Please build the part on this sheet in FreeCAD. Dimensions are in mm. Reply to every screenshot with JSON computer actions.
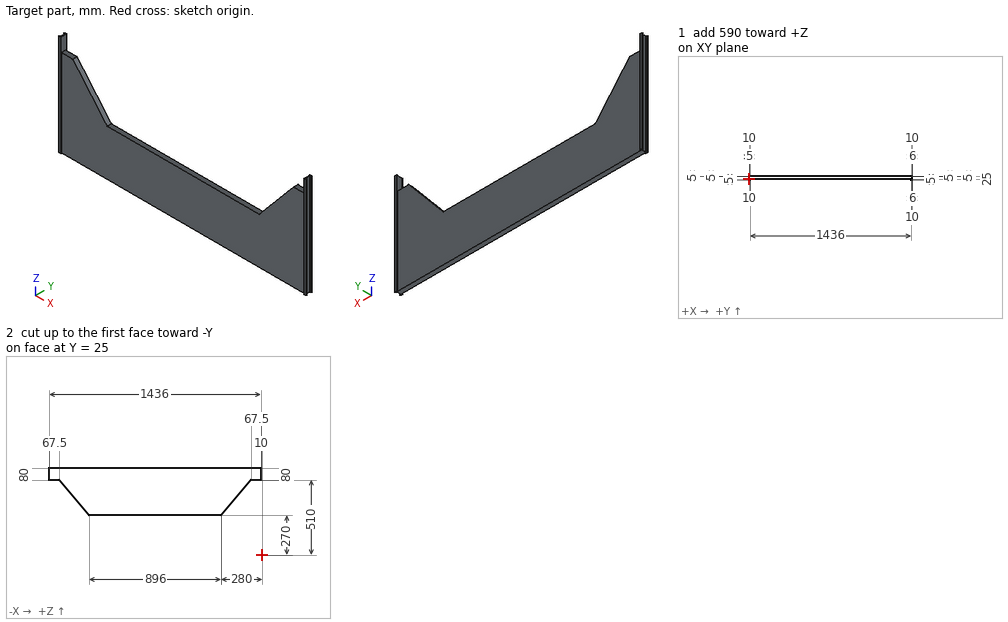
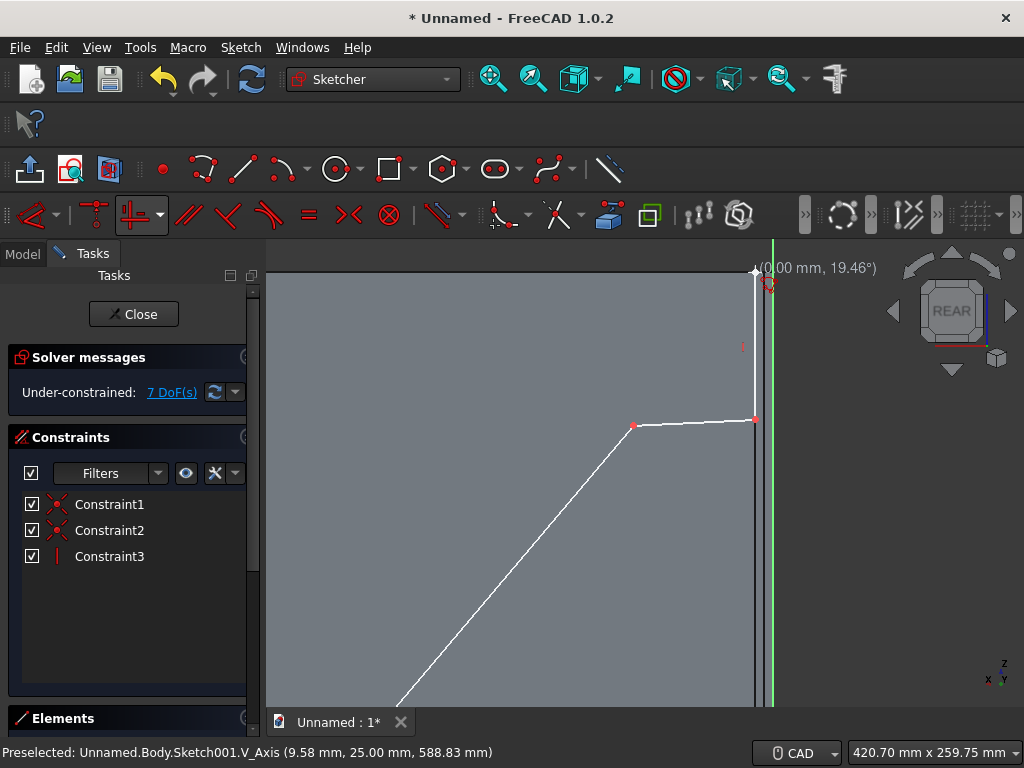
{"action": "scroll", "coordinate": [796, 408], "scroll_direction": "down", "scroll_amount": 9}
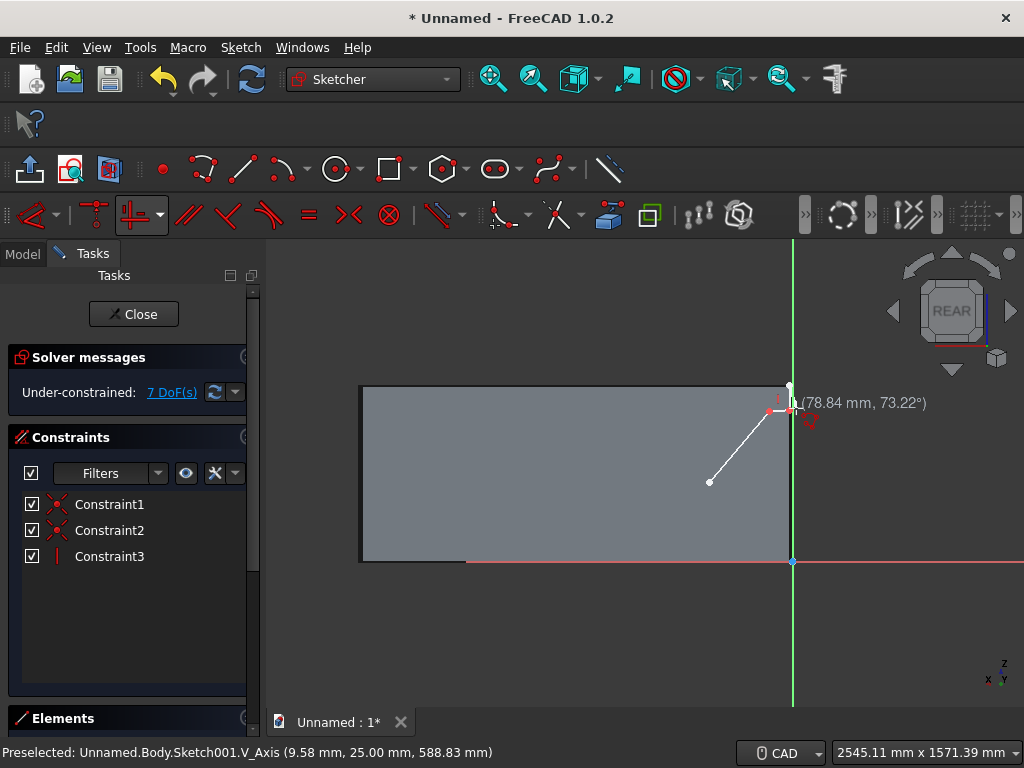
{"action": "left_click", "coordinate": [362, 386]}
{"action": "left_click", "coordinate": [362, 410]}
{"action": "left_click", "coordinate": [382, 410]}
{"action": "left_click", "coordinate": [443, 481]}
{"action": "left_click", "coordinate": [710, 482]}
{"action": "key", "text": "Escape"}
{"action": "key", "text": "Escape"}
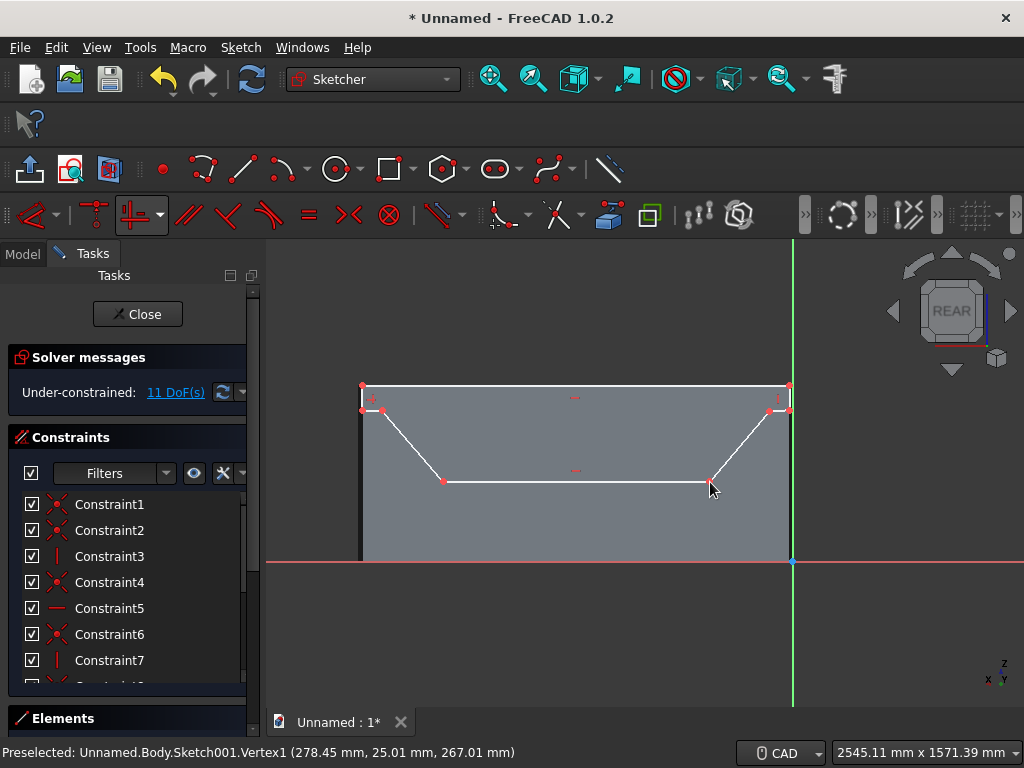
{"action": "scroll", "coordinate": [780, 411], "scroll_direction": "up", "scroll_amount": 2}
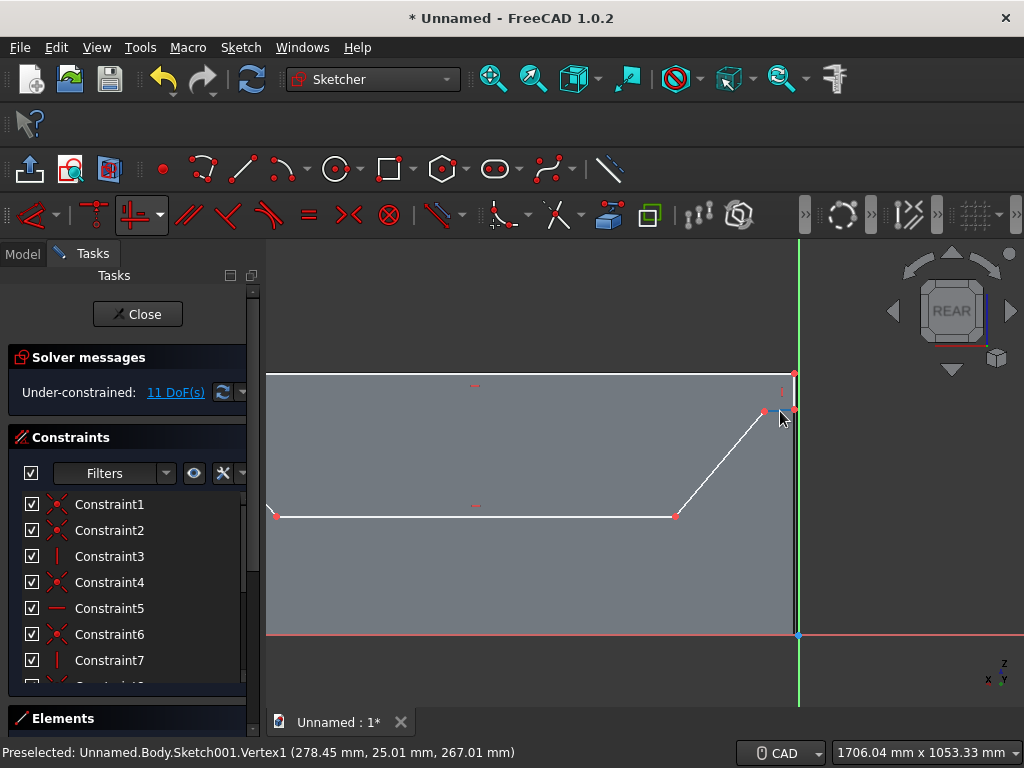
{"action": "left_click", "coordinate": [779, 410]}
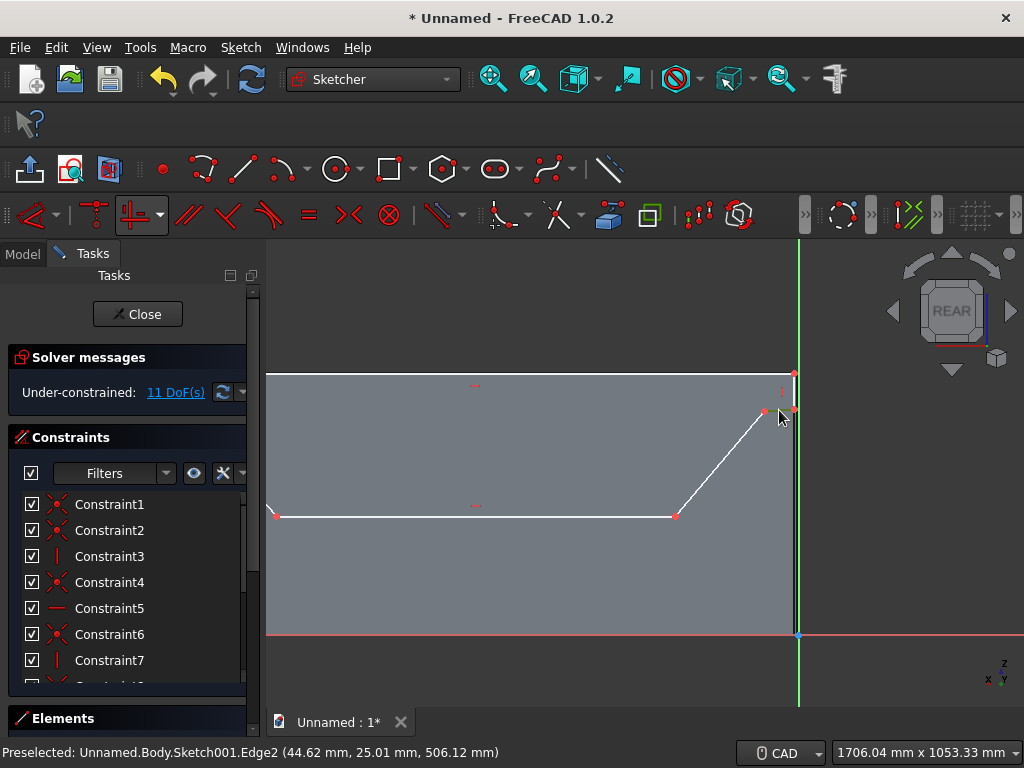
{"action": "key", "text": "h"}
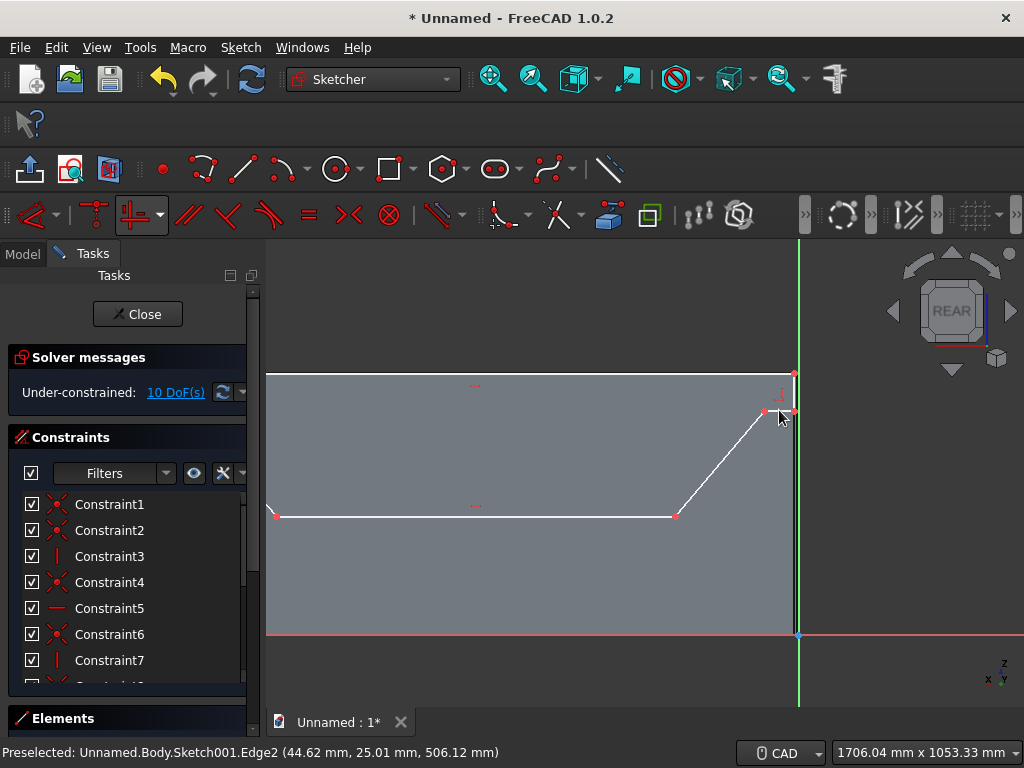
{"action": "left_click", "coordinate": [32, 216]}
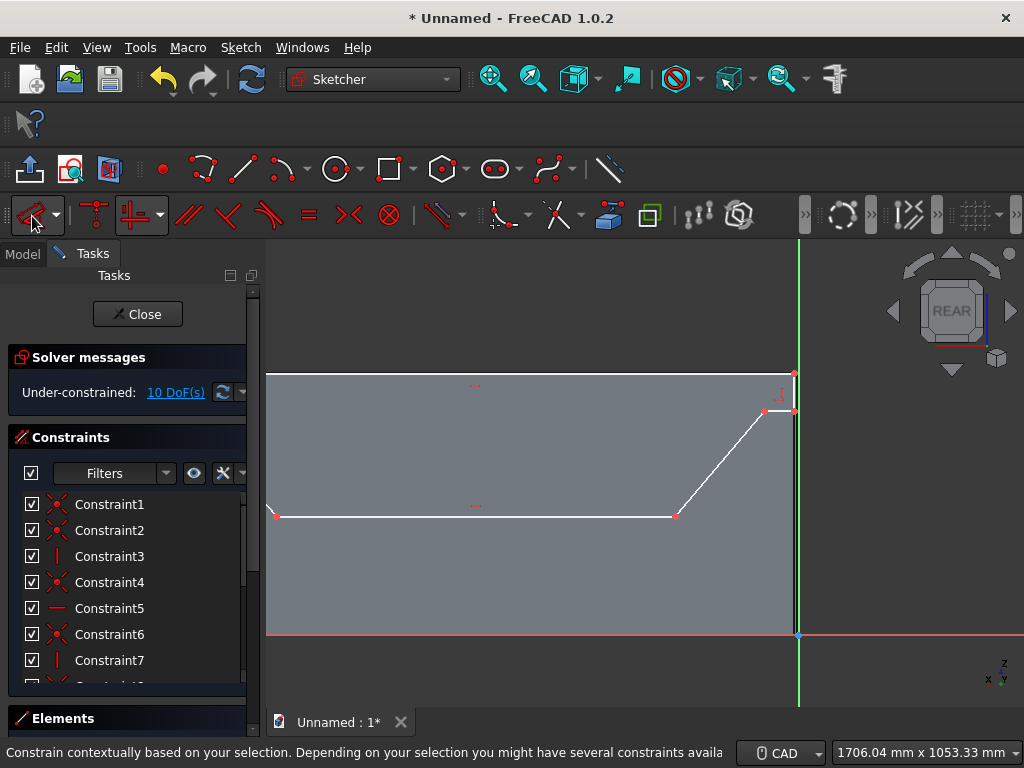
{"action": "scroll", "coordinate": [794, 400], "scroll_direction": "up", "scroll_amount": 6}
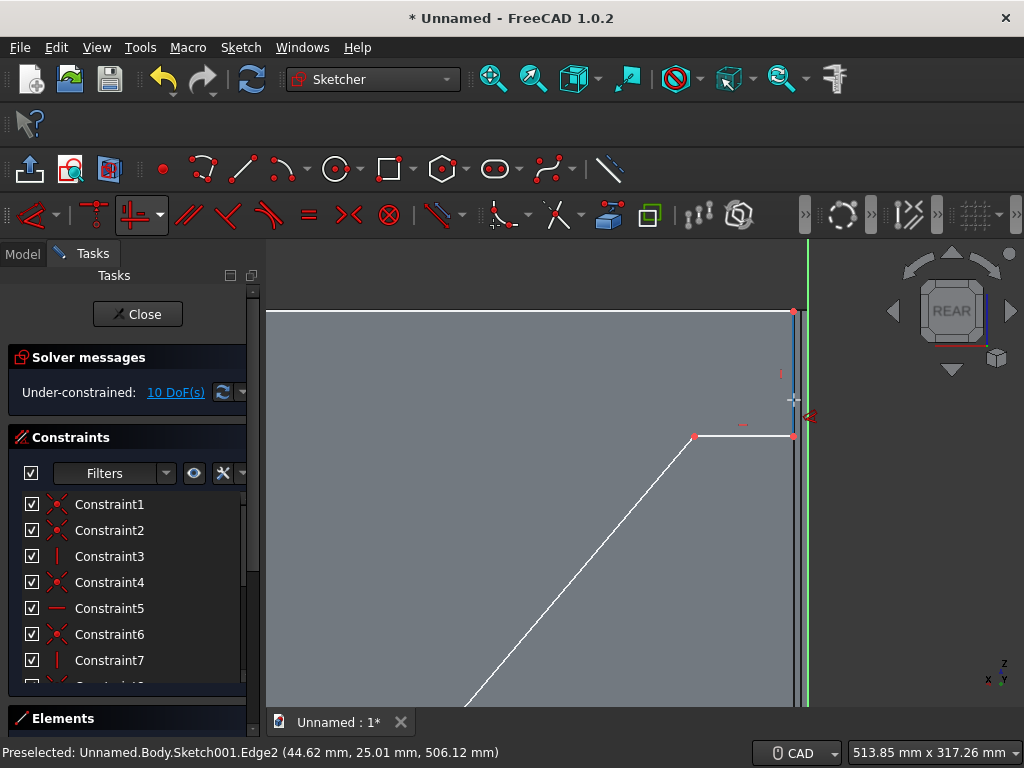
{"action": "left_click", "coordinate": [793, 399]}
{"action": "left_click", "coordinate": [827, 374]}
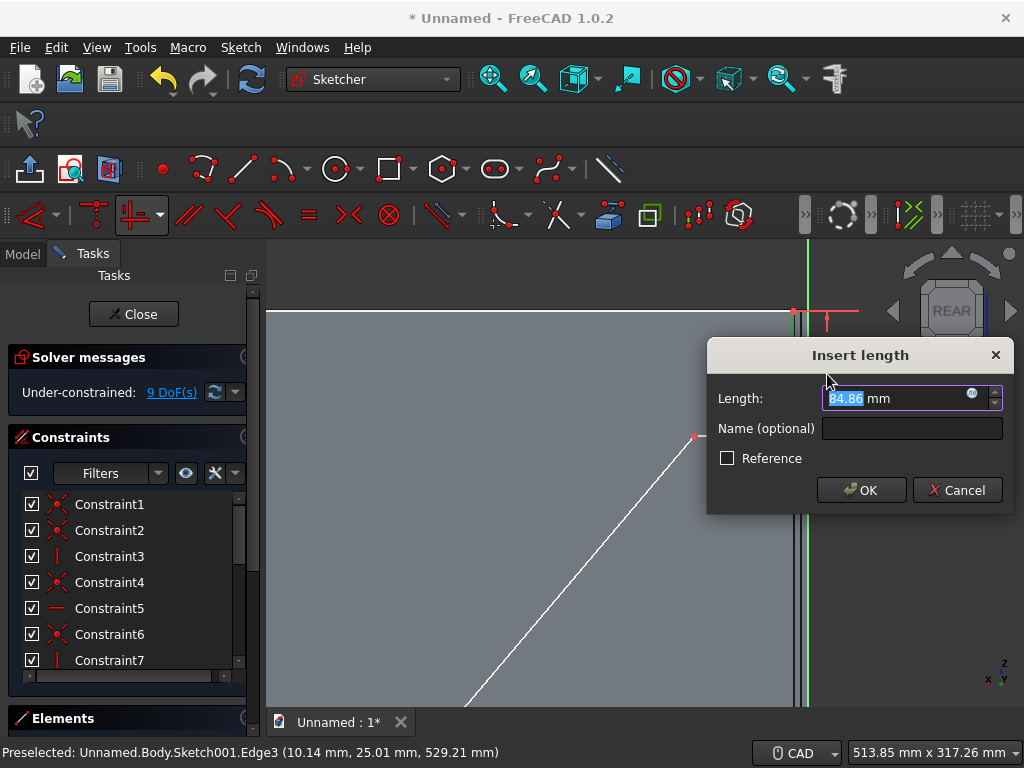
{"action": "type", "text": "80"}
{"action": "key", "text": "Return"}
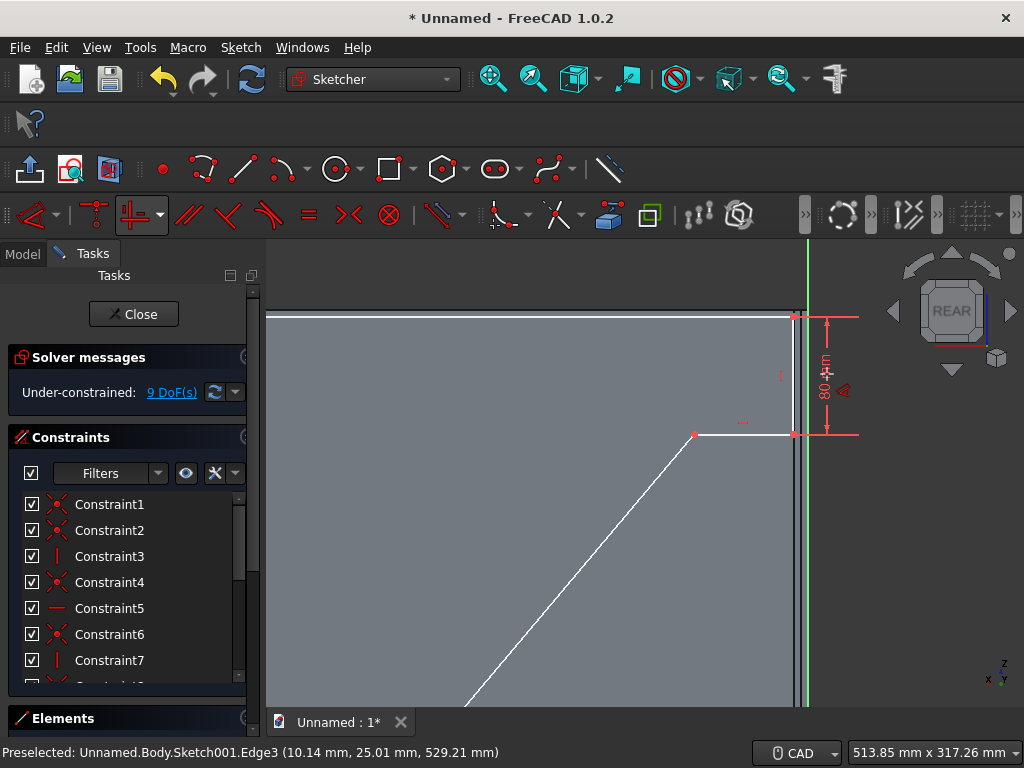
{"action": "scroll", "coordinate": [788, 404], "scroll_direction": "down", "scroll_amount": 8}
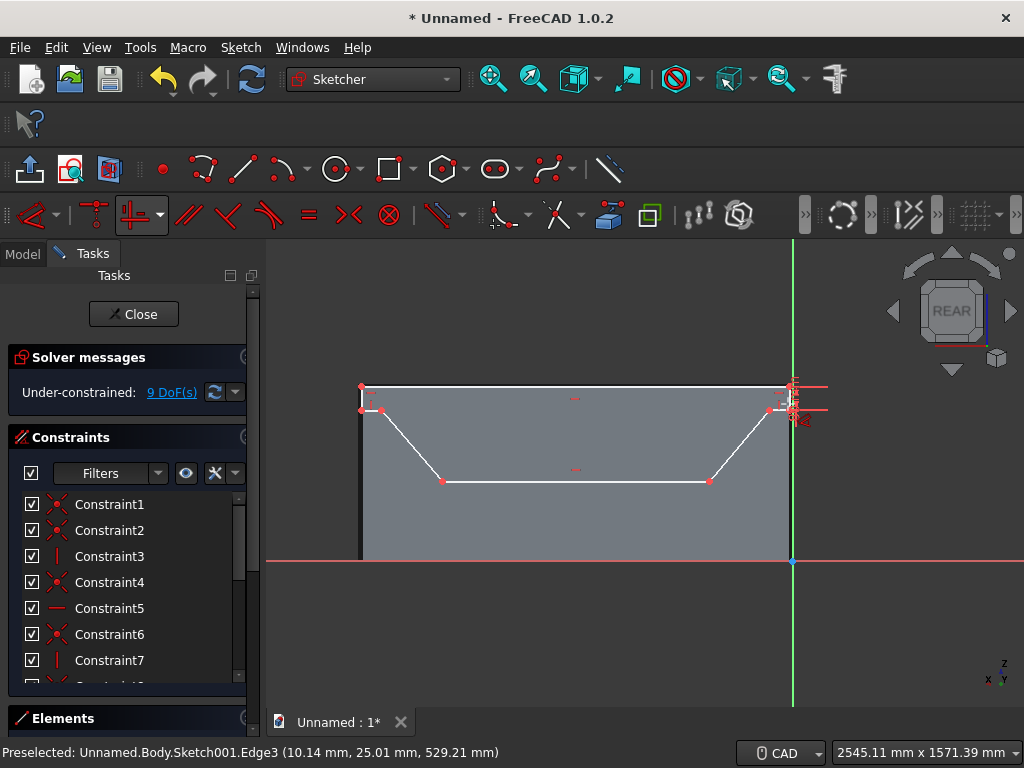
{"action": "scroll", "coordinate": [362, 394], "scroll_direction": "up", "scroll_amount": 4}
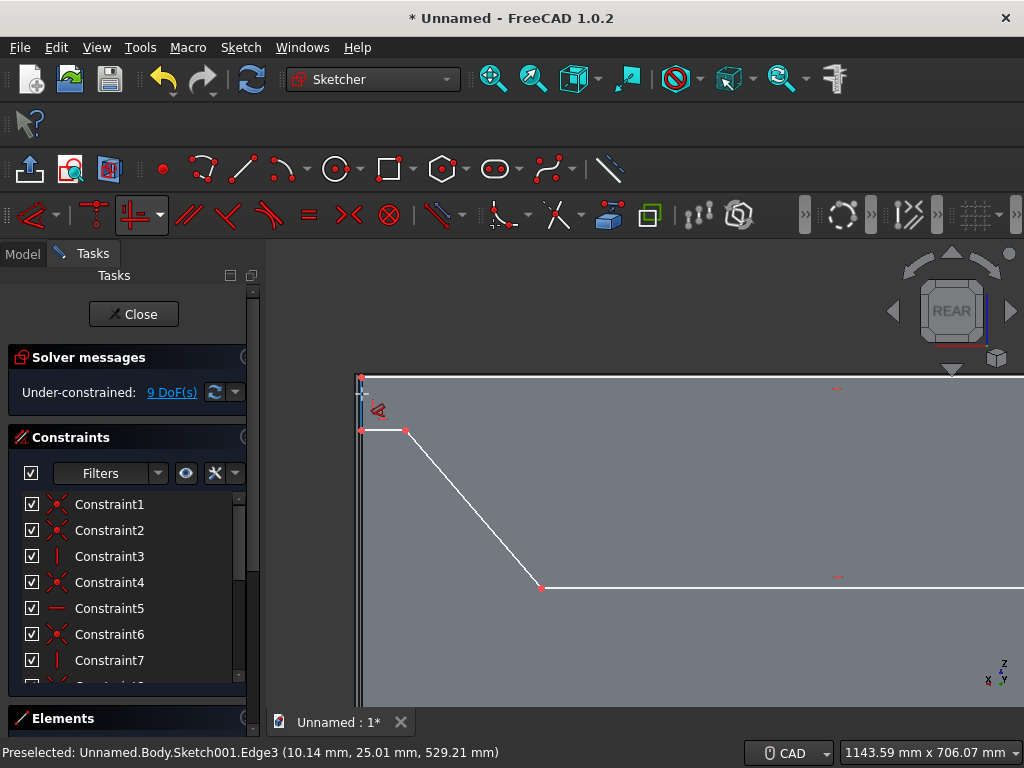
{"action": "left_click", "coordinate": [361, 393]}
{"action": "left_click", "coordinate": [327, 404]}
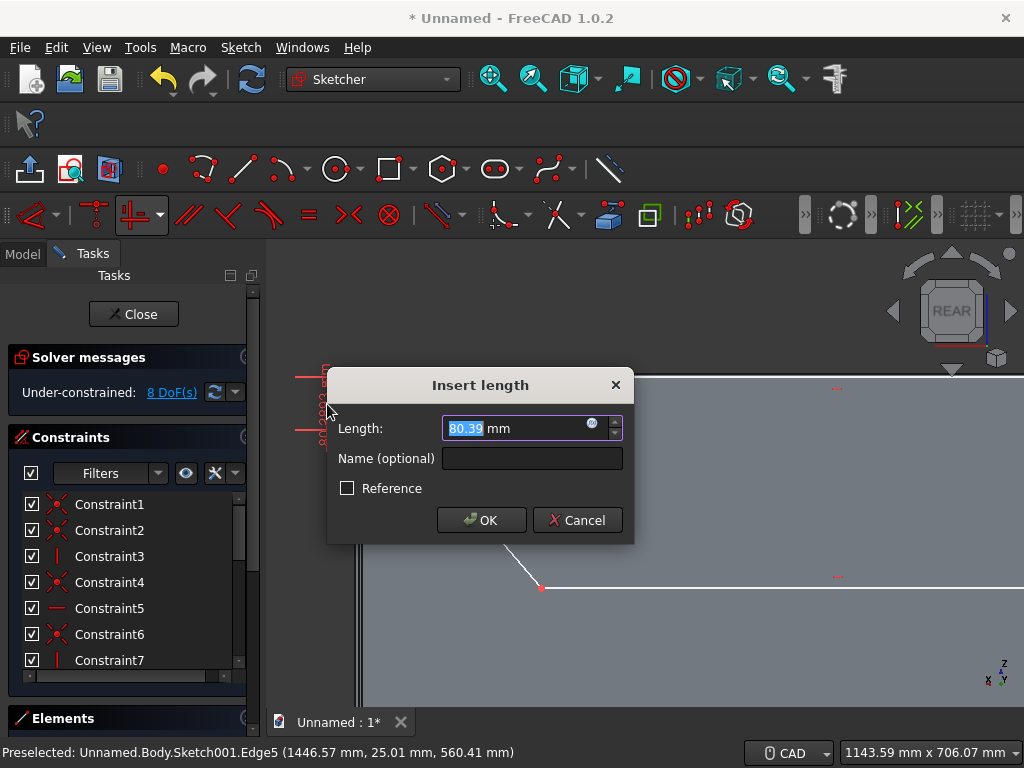
{"action": "type", "text": "80"}
{"action": "key", "text": "Return"}